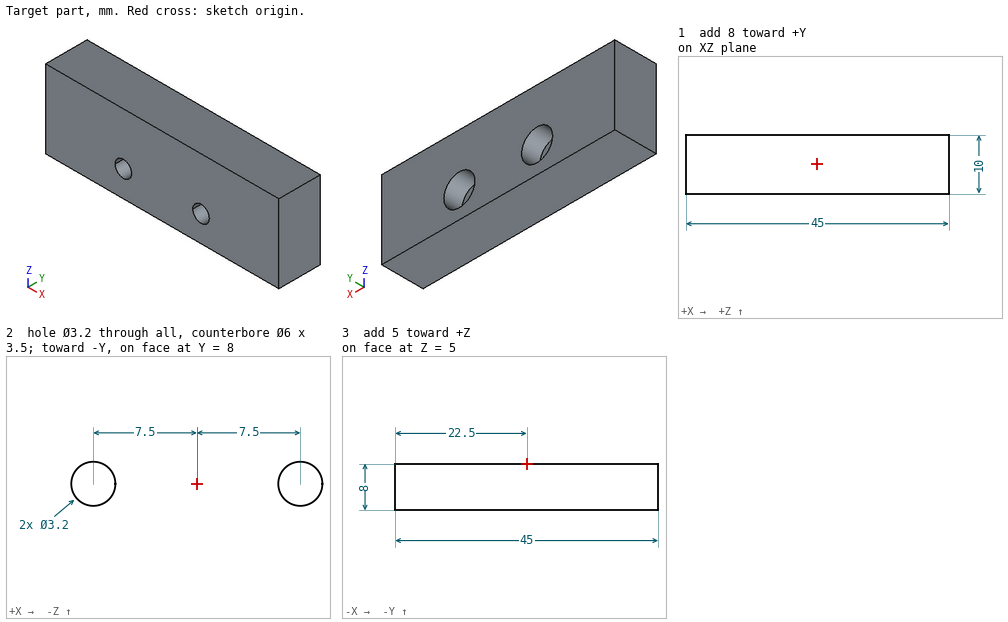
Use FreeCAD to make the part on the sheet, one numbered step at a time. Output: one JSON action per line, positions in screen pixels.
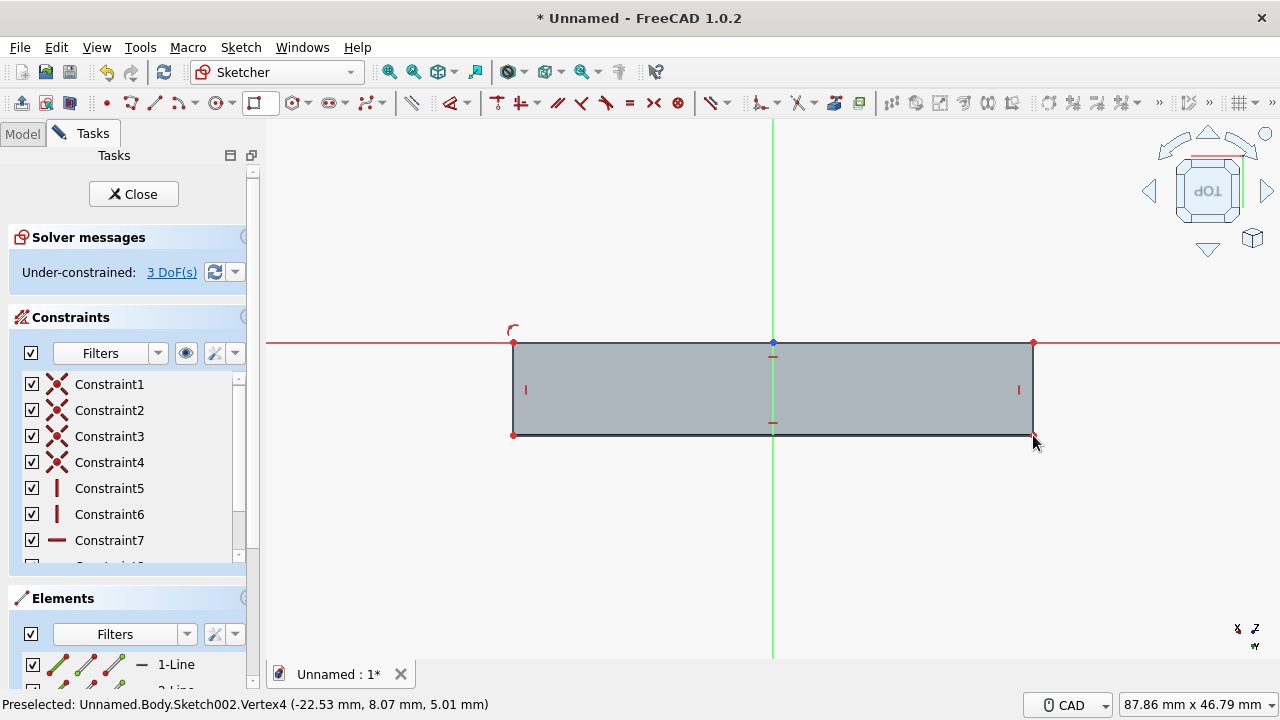
{"action": "left_click", "coordinate": [450, 104]}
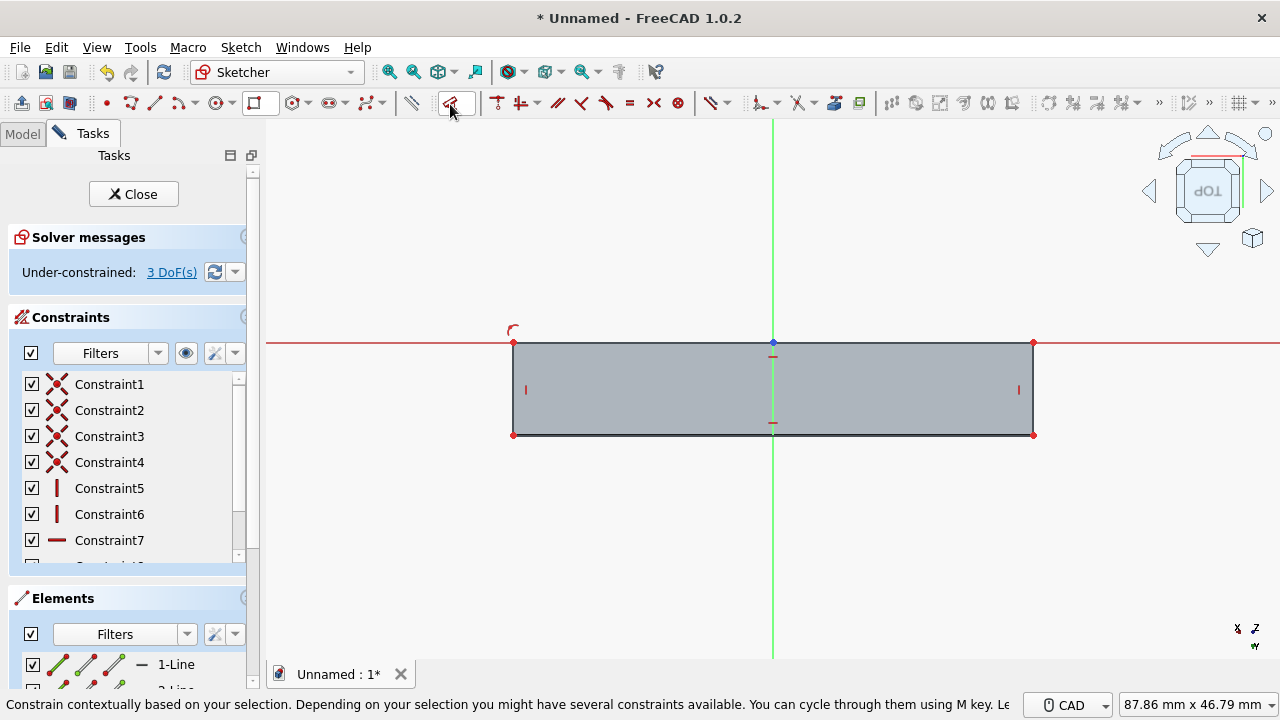
{"action": "left_click", "coordinate": [513, 371]}
{"action": "left_click", "coordinate": [479, 389]}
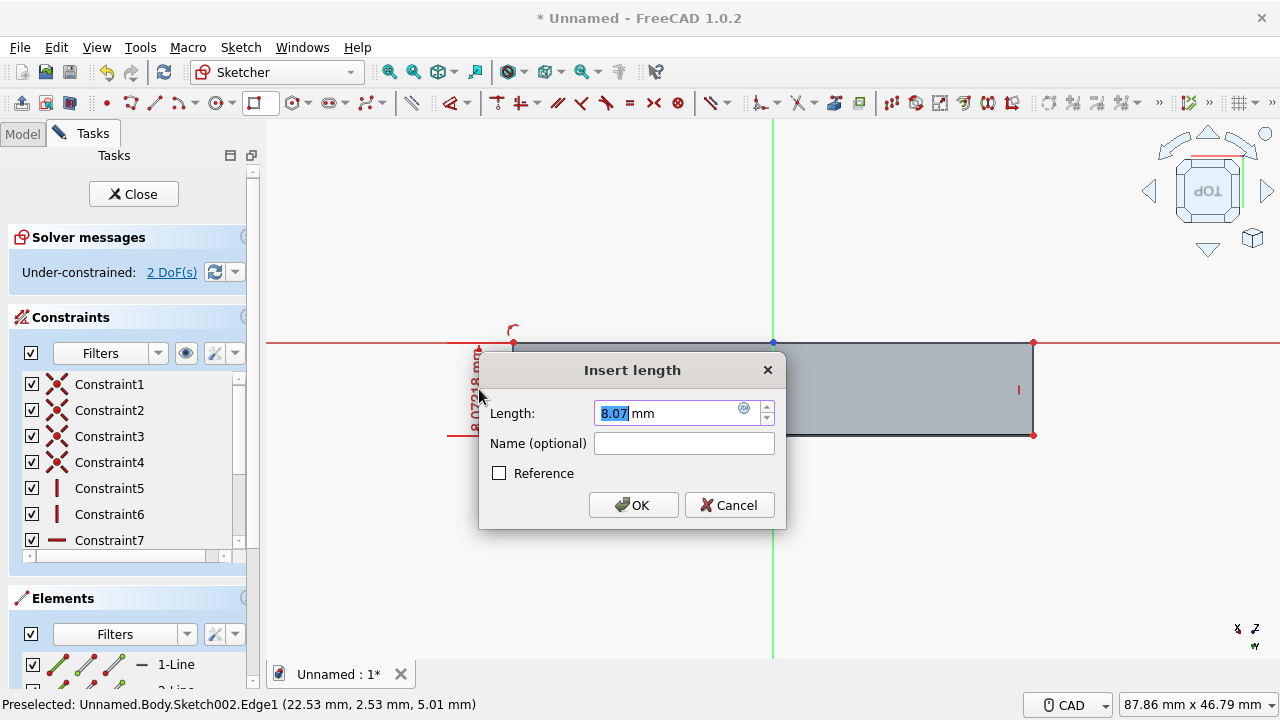
{"action": "type", "text": "8"}
{"action": "key", "text": "Return"}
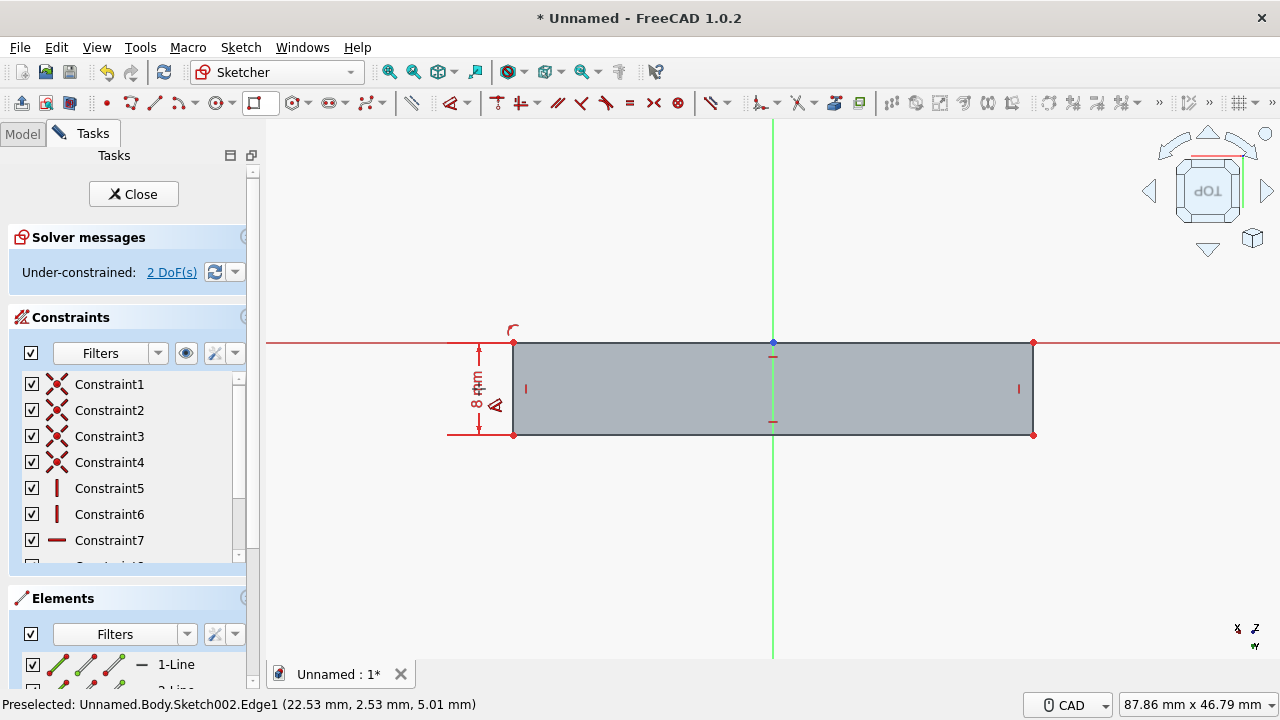
{"action": "left_click", "coordinate": [669, 435]}
{"action": "left_click", "coordinate": [653, 469]}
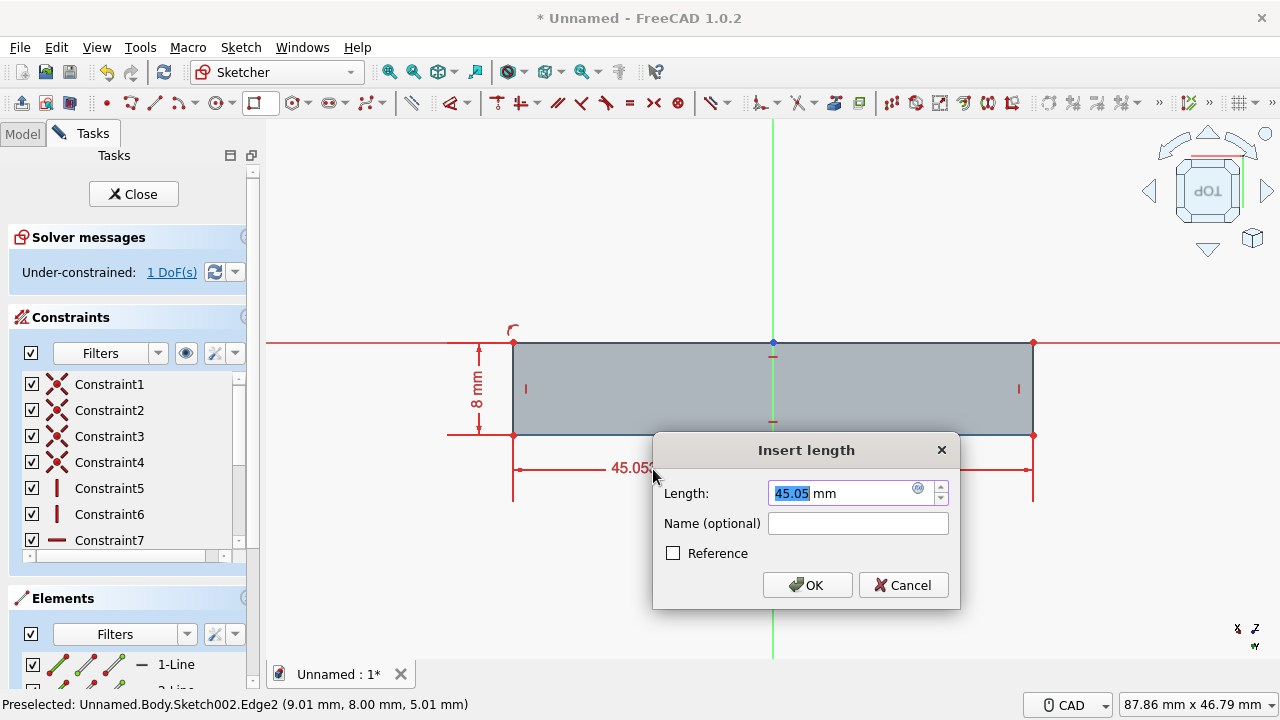
{"action": "type", "text": "45"}
{"action": "key", "text": "Return"}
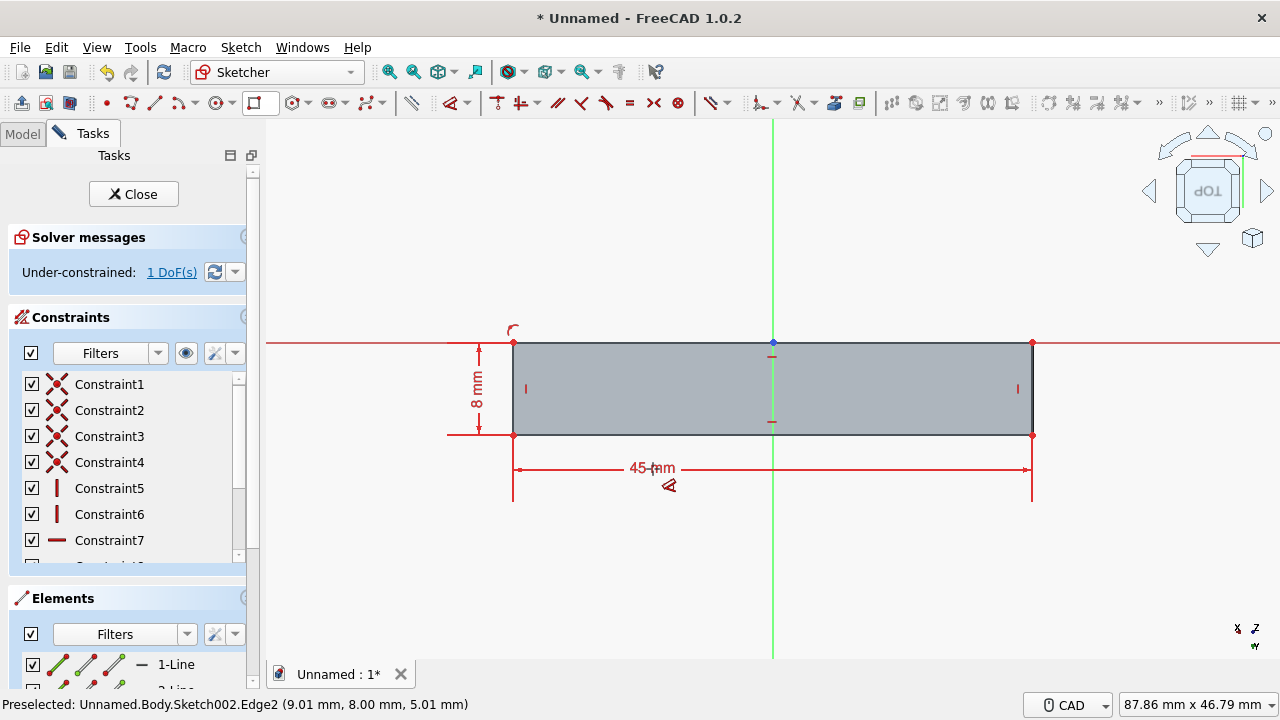
{"action": "left_click", "coordinate": [513, 343]}
{"action": "left_click", "coordinate": [643, 309]}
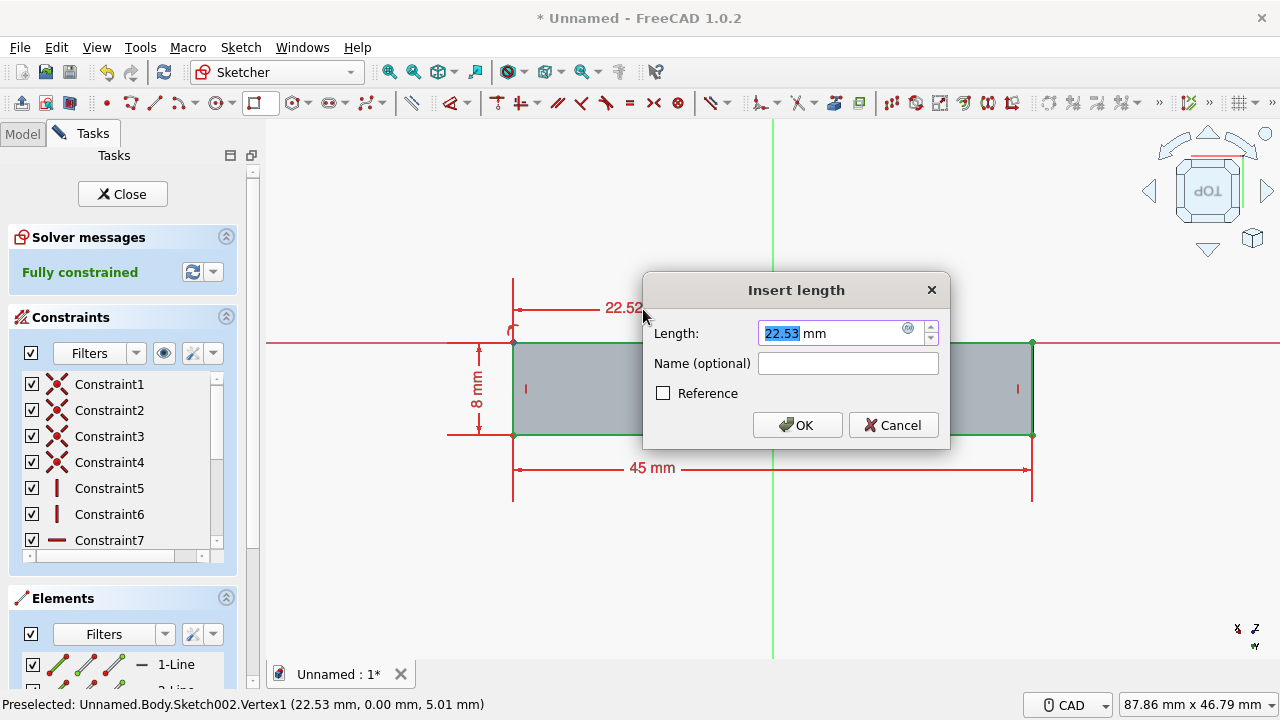
{"action": "type", "text": "22.5"}
{"action": "key", "text": "Return"}
{"action": "key", "text": "Escape"}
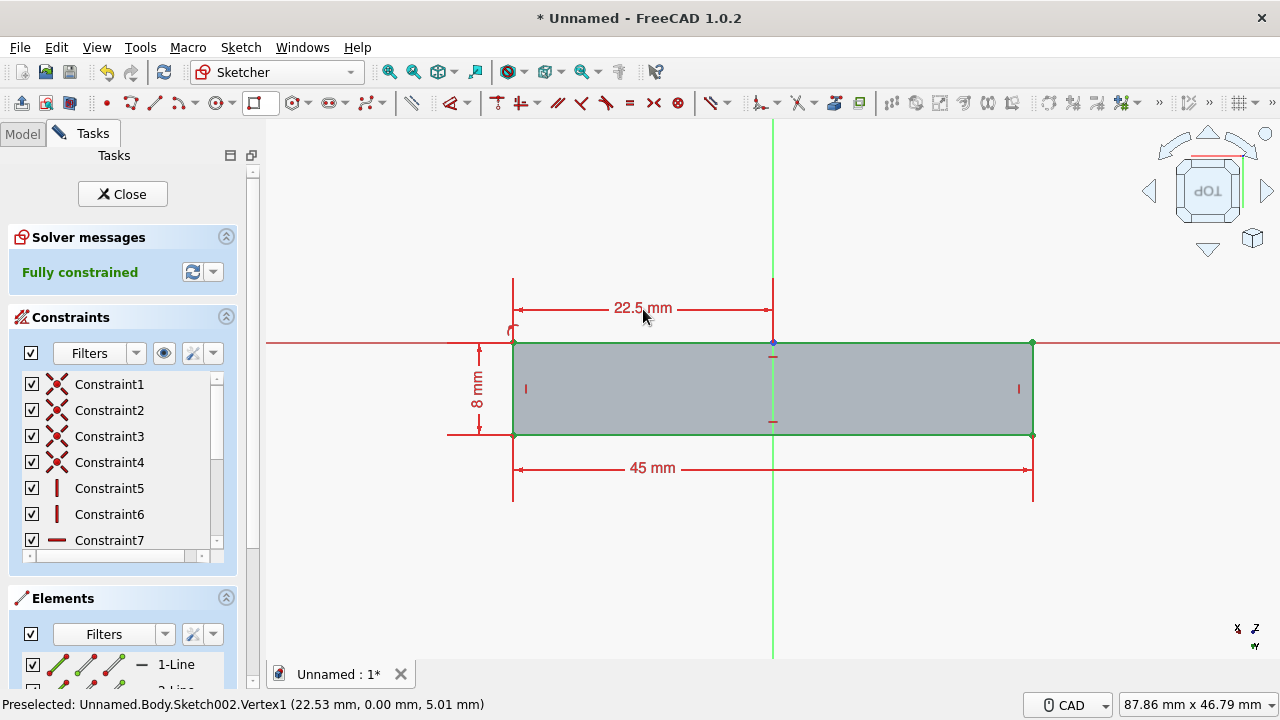
{"action": "left_click", "coordinate": [123, 194]}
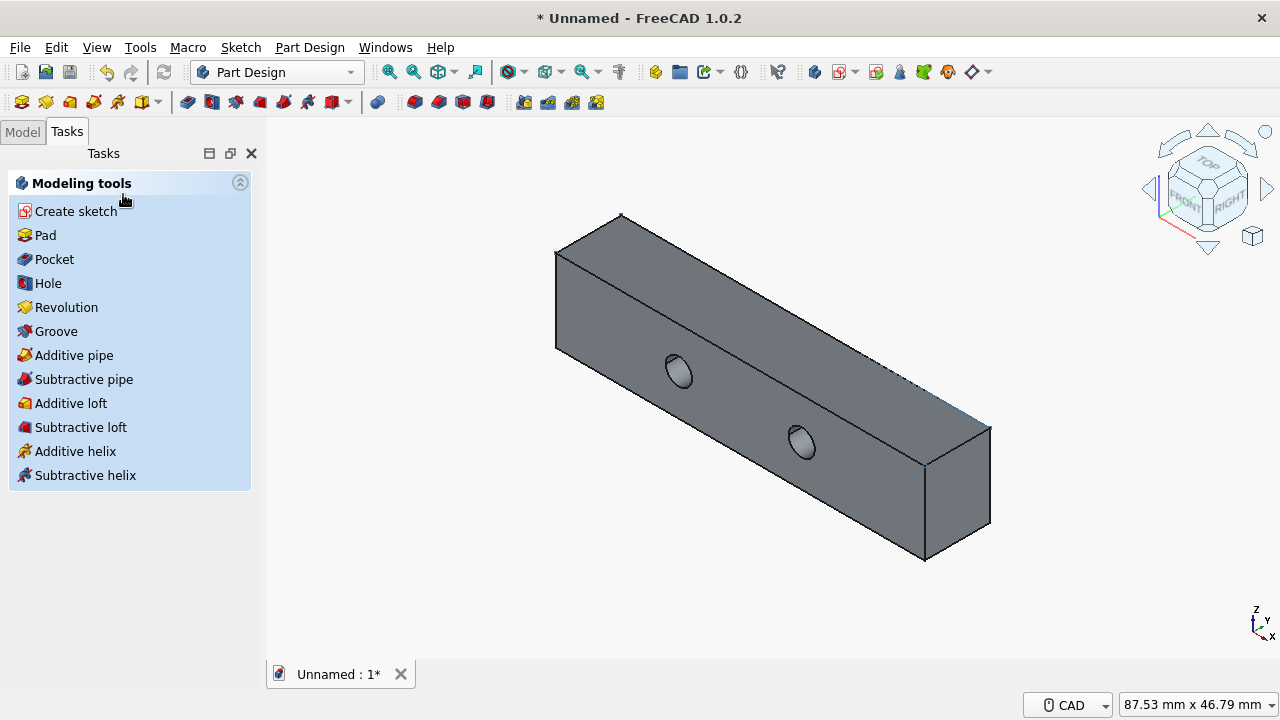
{"action": "left_click", "coordinate": [22, 102]}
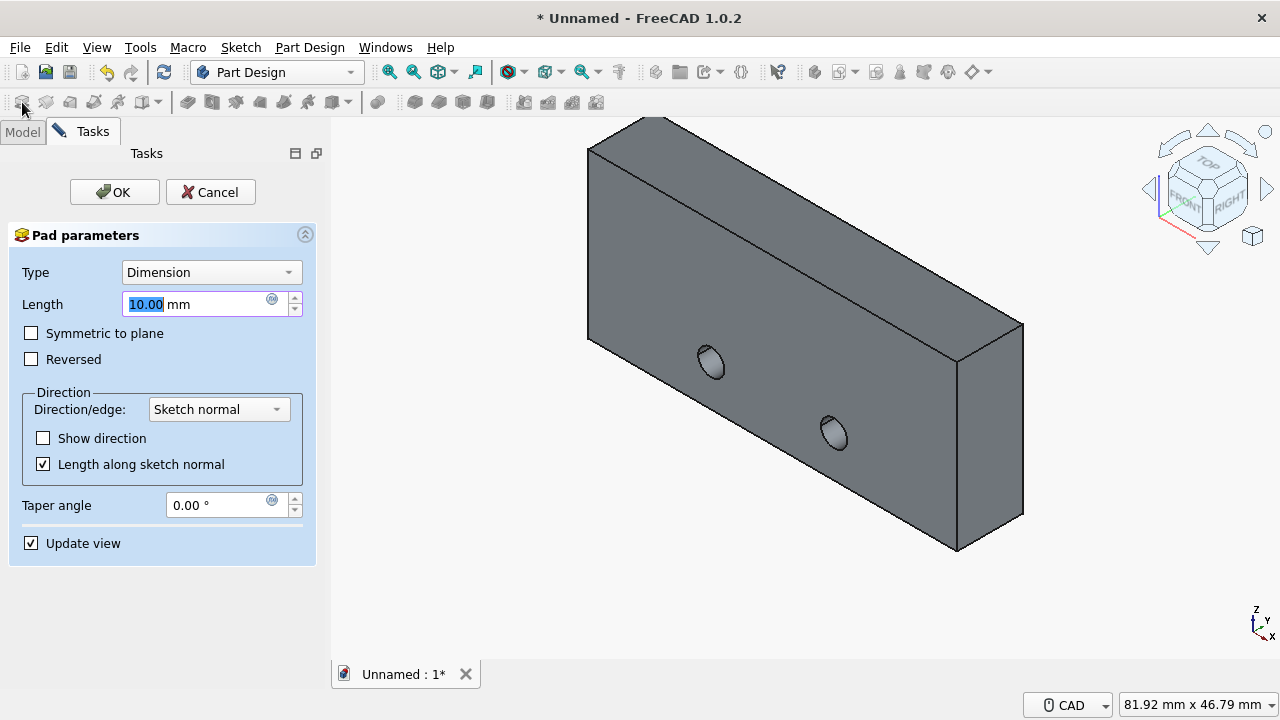
{"action": "type", "text": "5"}
{"action": "key", "text": "Tab"}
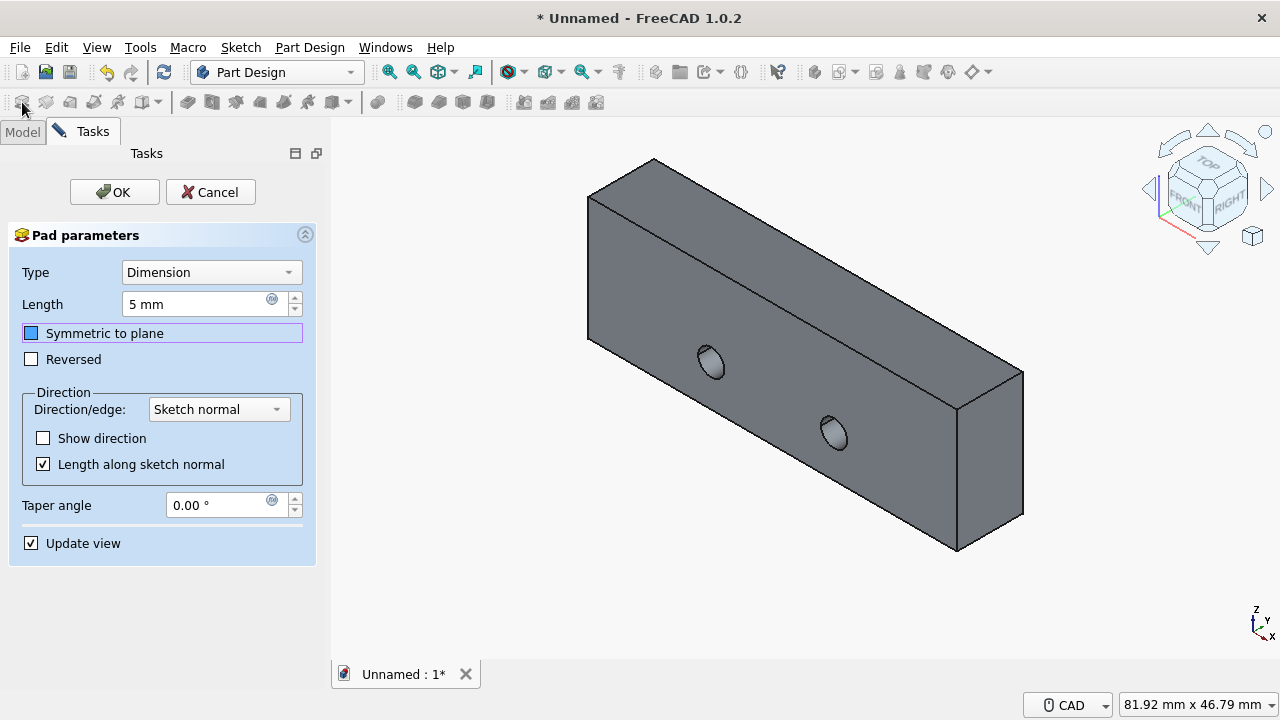
{"action": "left_click", "coordinate": [115, 192]}